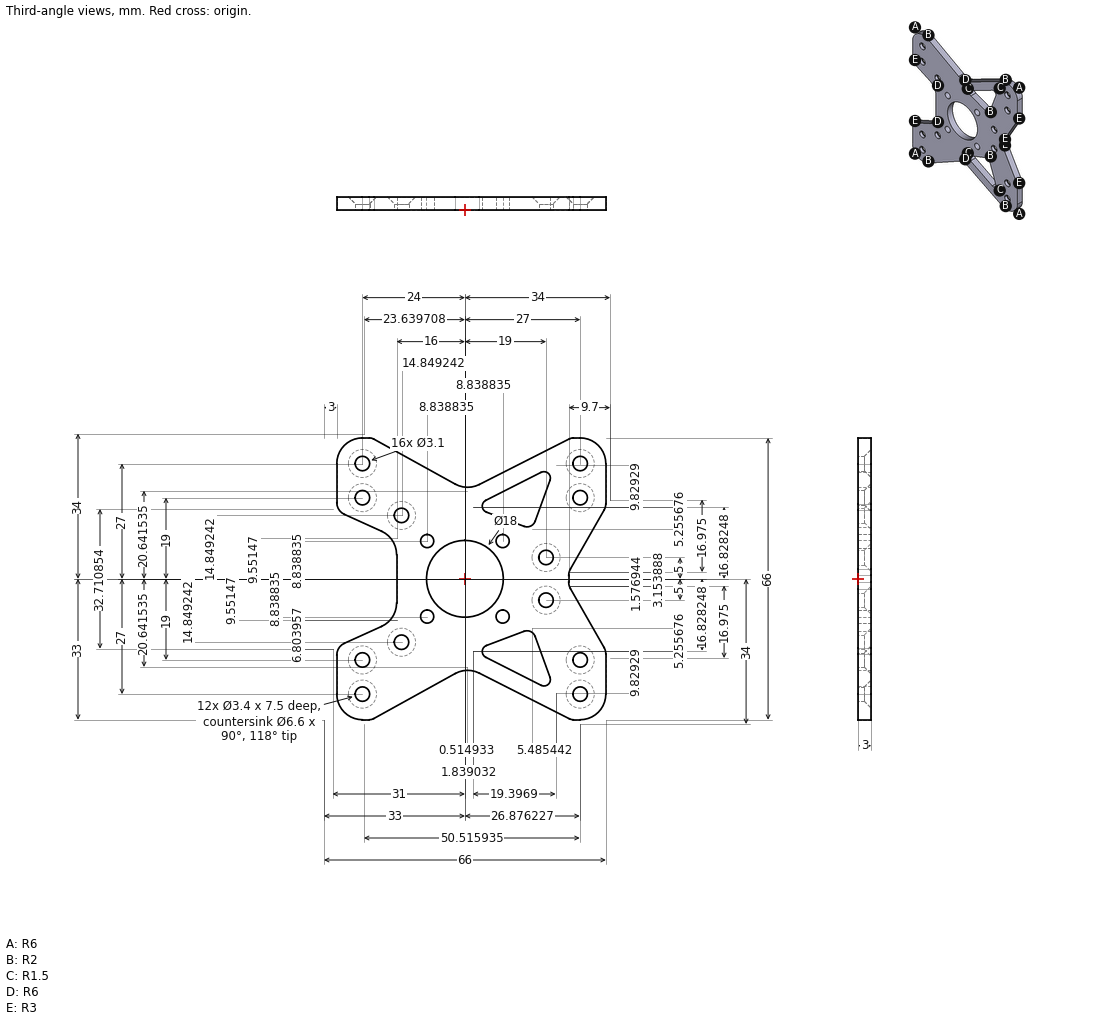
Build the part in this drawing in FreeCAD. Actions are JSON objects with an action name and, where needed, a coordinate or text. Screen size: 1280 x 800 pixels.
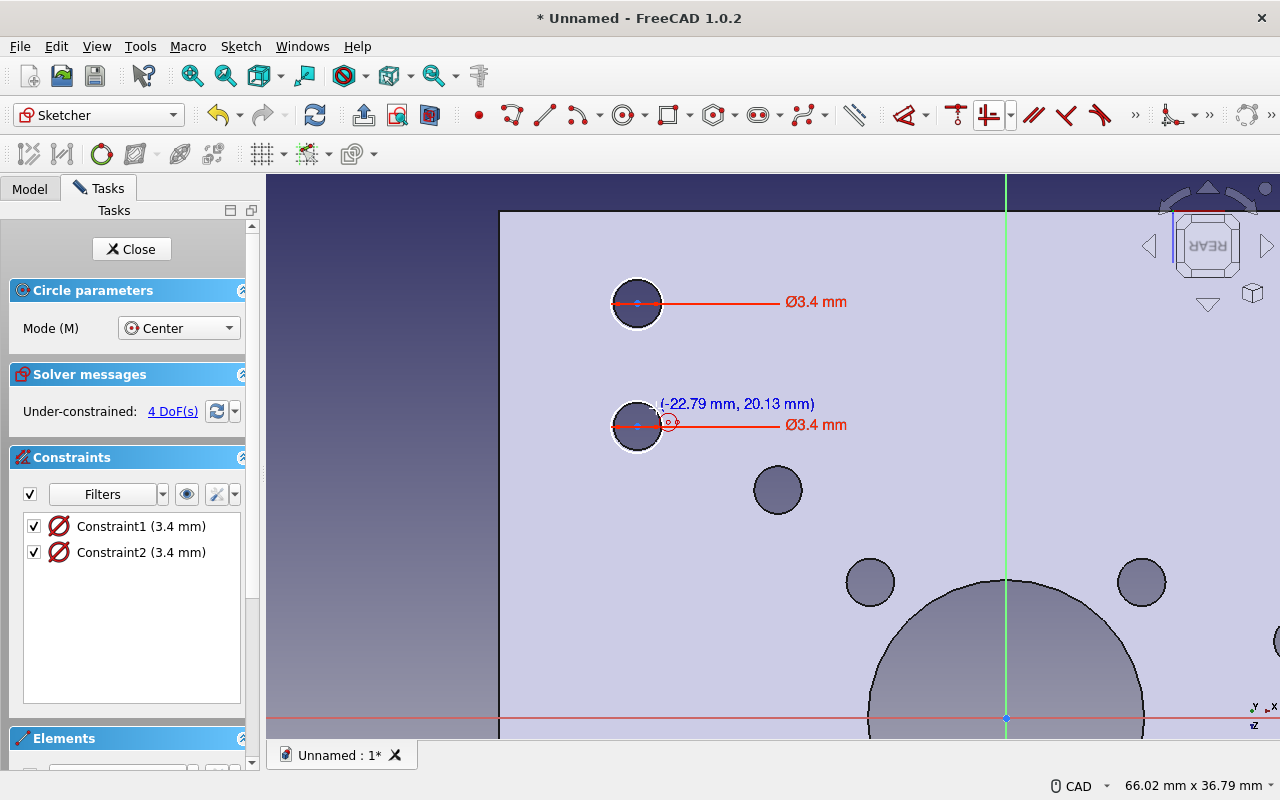
{"action": "scroll", "coordinate": [440, 243], "scroll_direction": "down", "scroll_amount": 4}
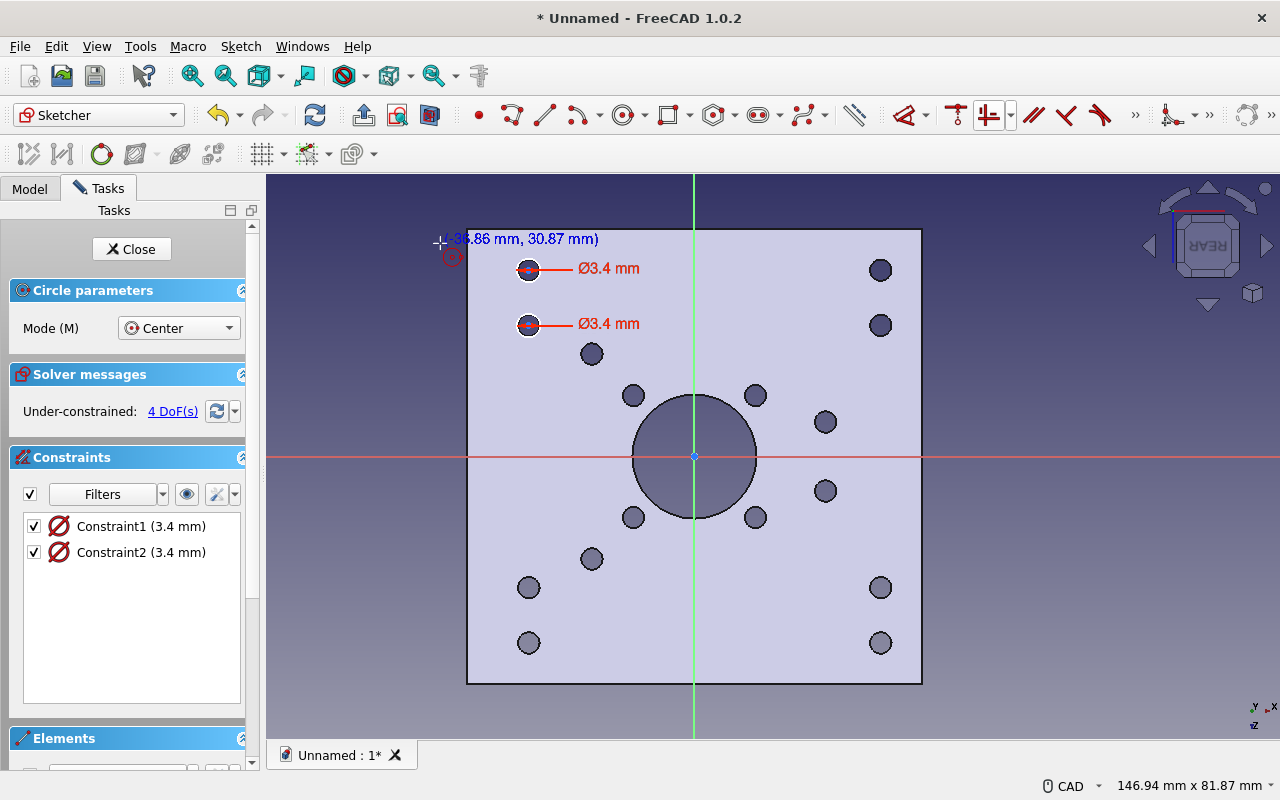
{"action": "scroll", "coordinate": [529, 588], "scroll_direction": "up", "scroll_amount": 4}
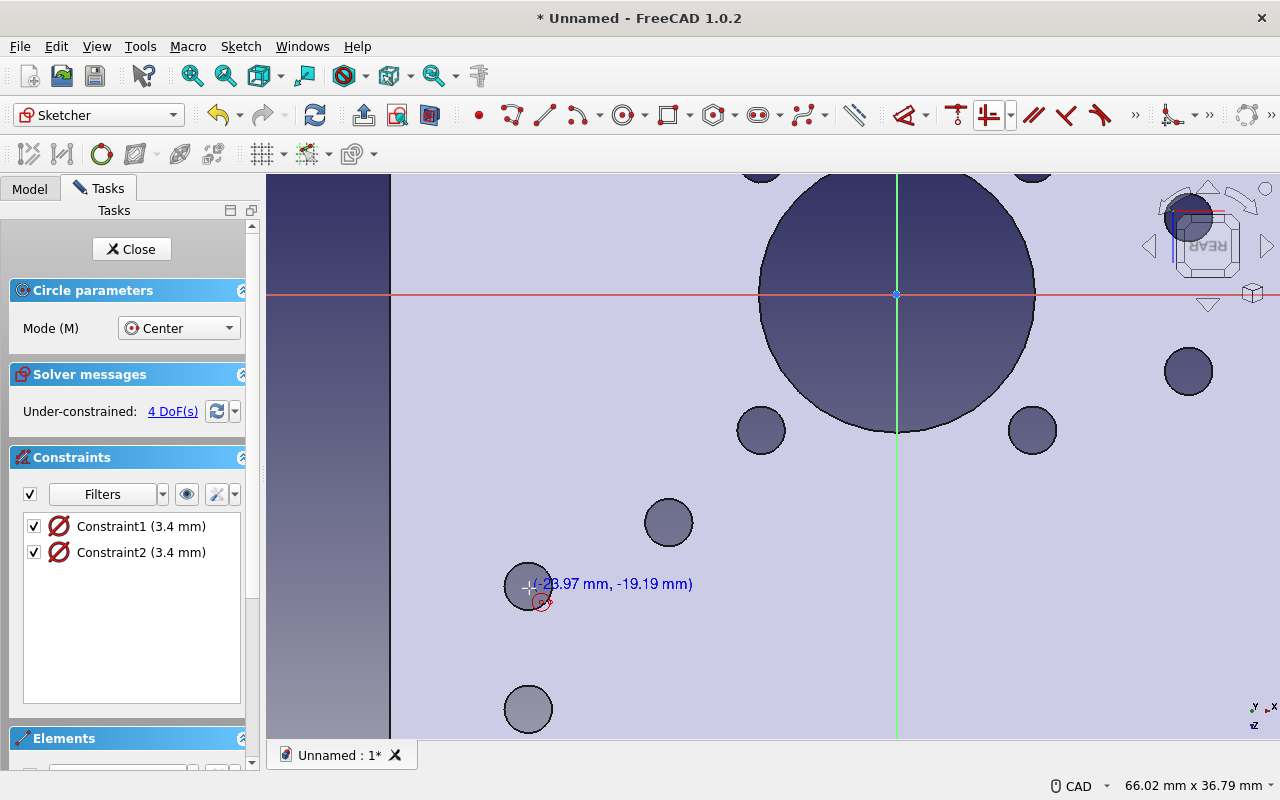
{"action": "left_click", "coordinate": [528, 586]}
{"action": "mouse_move", "coordinate": [547, 568]}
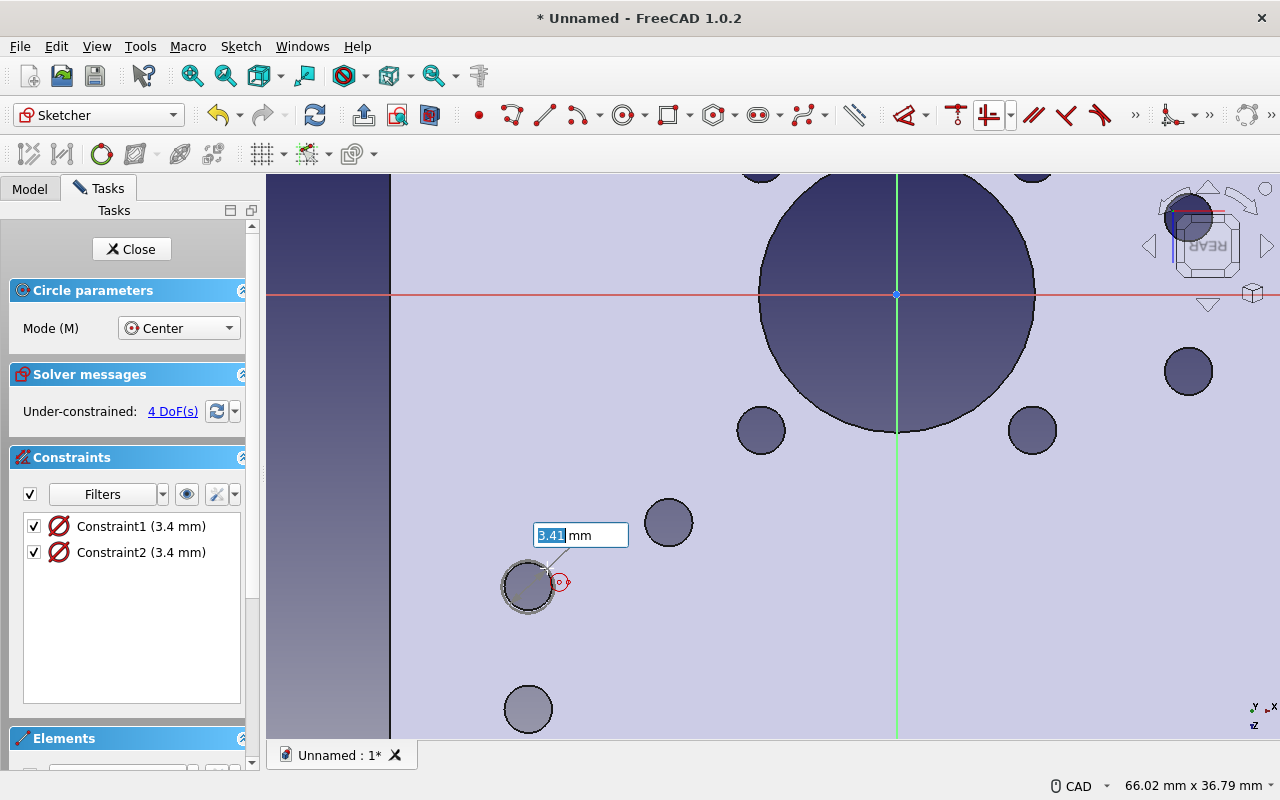
{"action": "type", "text": "3.4"}
{"action": "key", "text": "Return"}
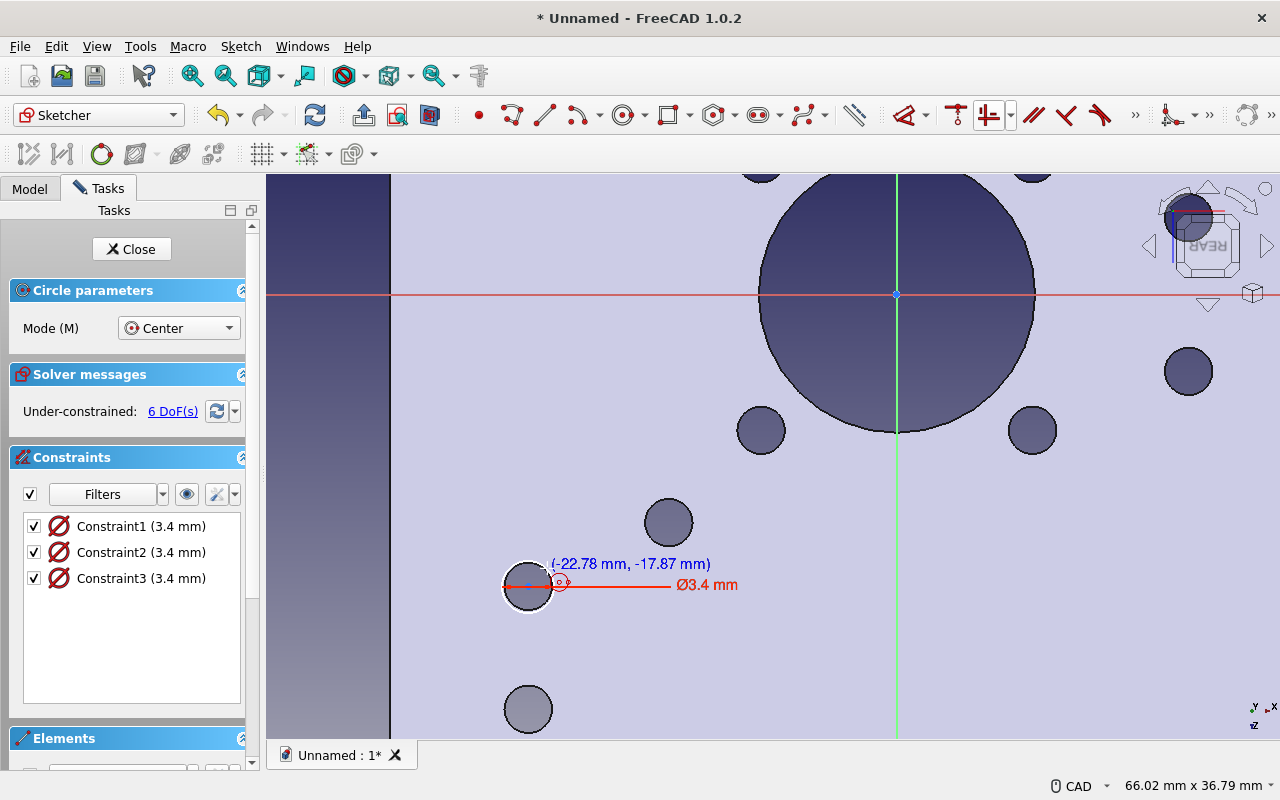
{"action": "left_click", "coordinate": [528, 709]}
{"action": "mouse_move", "coordinate": [547, 691]}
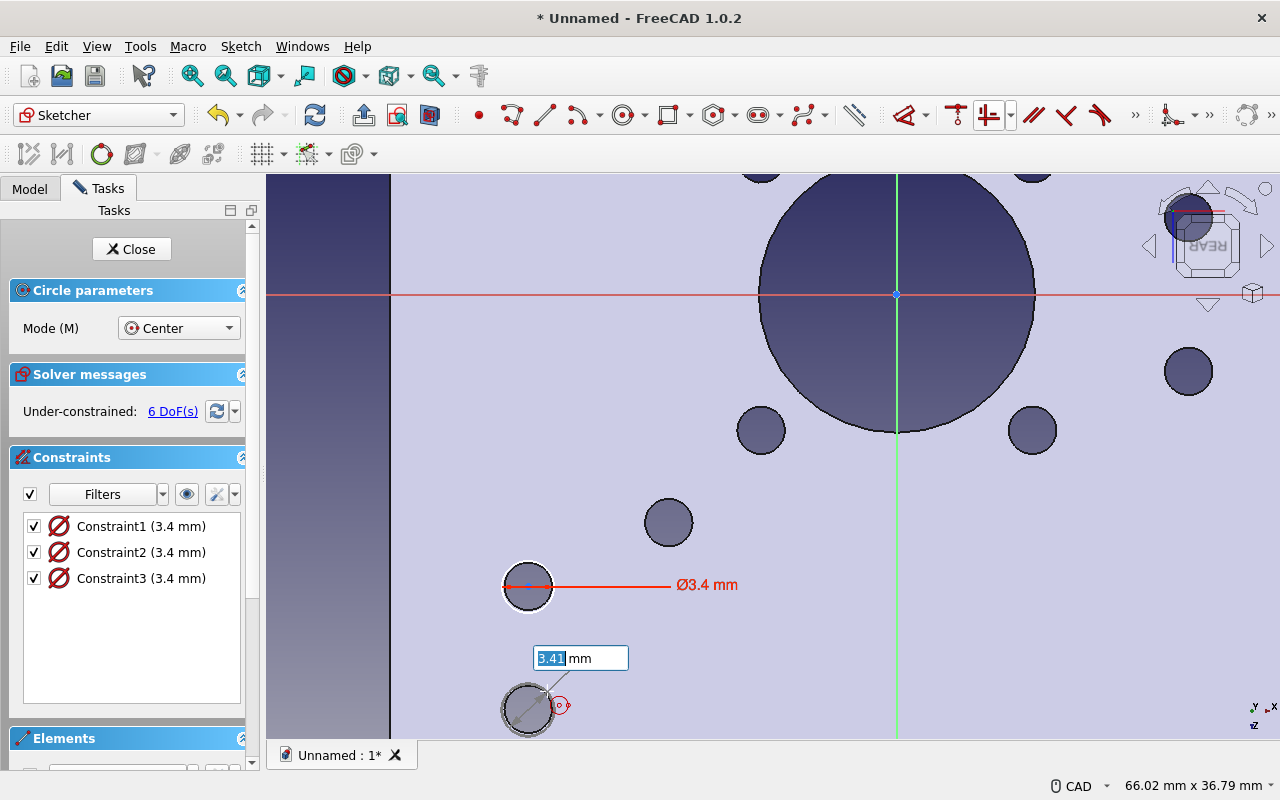
{"action": "type", "text": "3.4"}
{"action": "key", "text": "Return"}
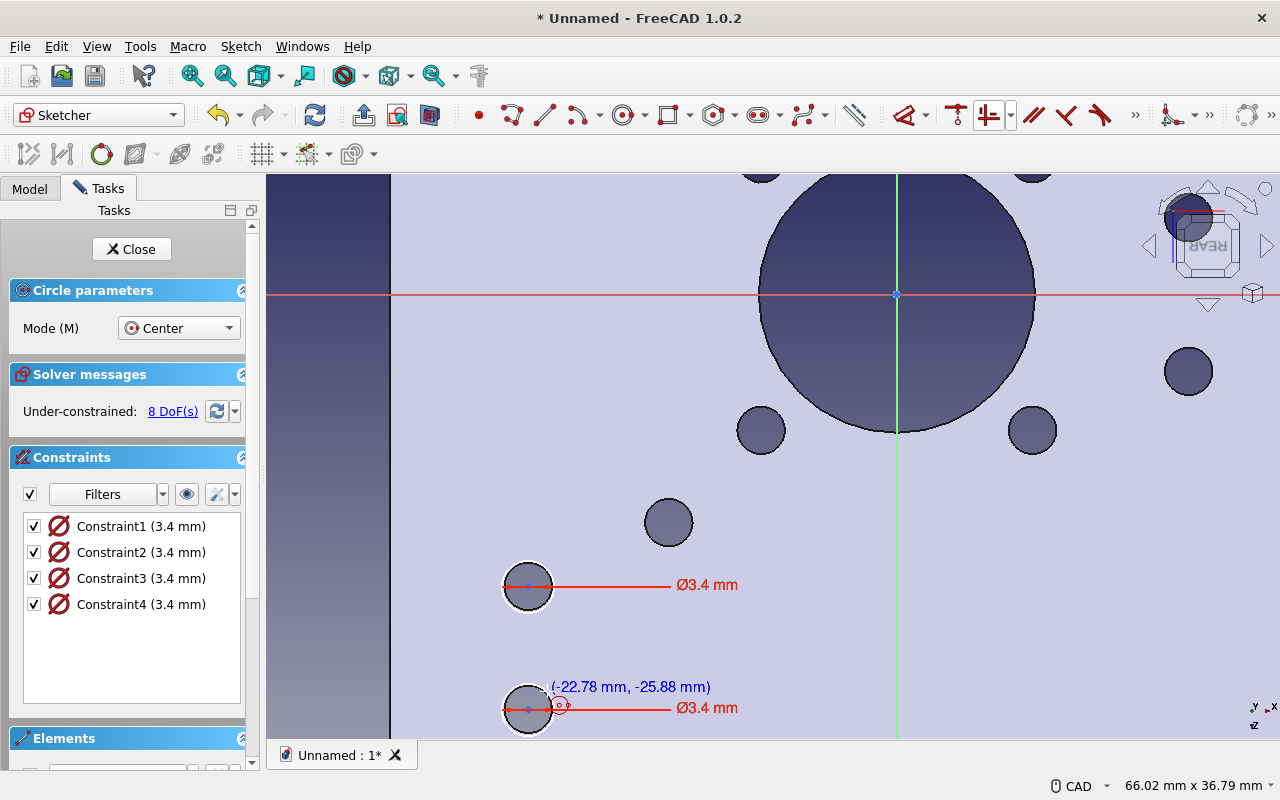
{"action": "scroll", "coordinate": [529, 589], "scroll_direction": "down", "scroll_amount": 4}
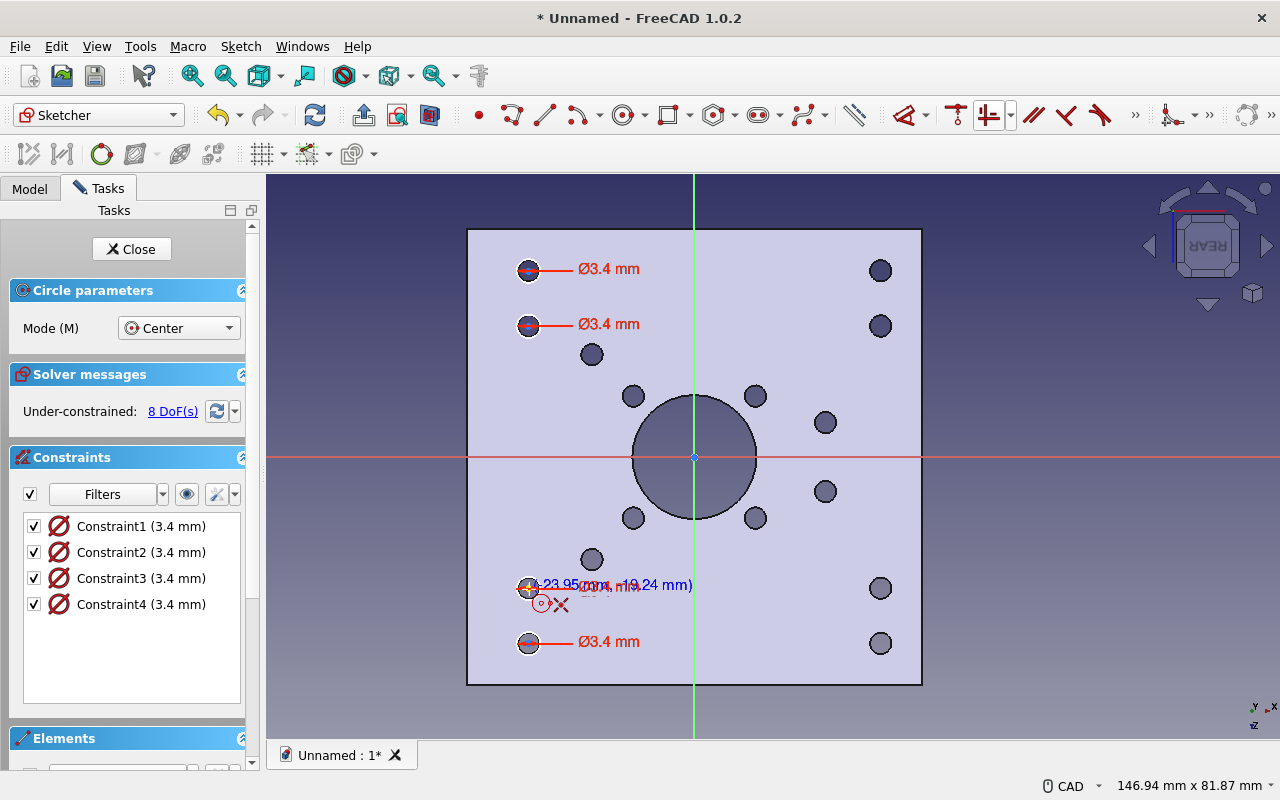
{"action": "scroll", "coordinate": [592, 355], "scroll_direction": "up", "scroll_amount": 4}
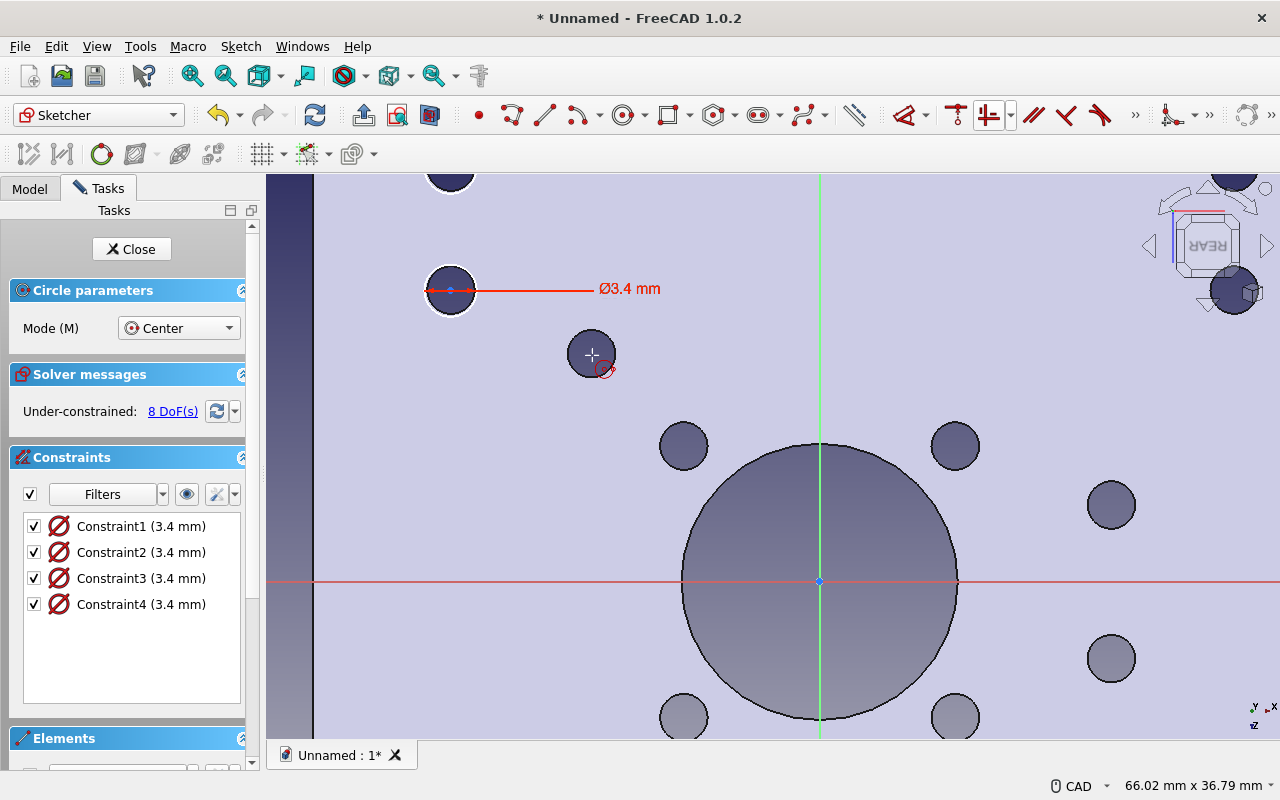
{"action": "left_click", "coordinate": [592, 354]}
{"action": "mouse_move", "coordinate": [610, 335]}